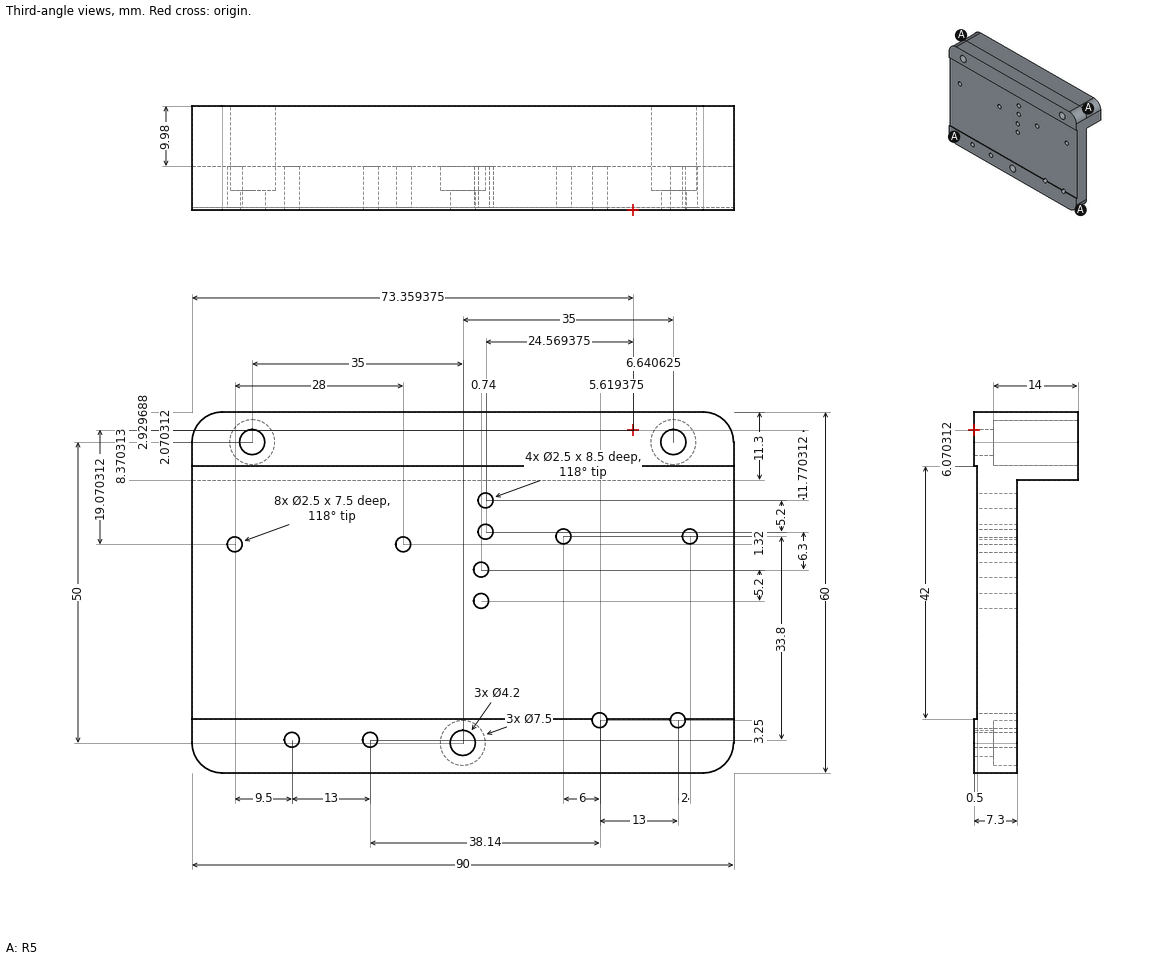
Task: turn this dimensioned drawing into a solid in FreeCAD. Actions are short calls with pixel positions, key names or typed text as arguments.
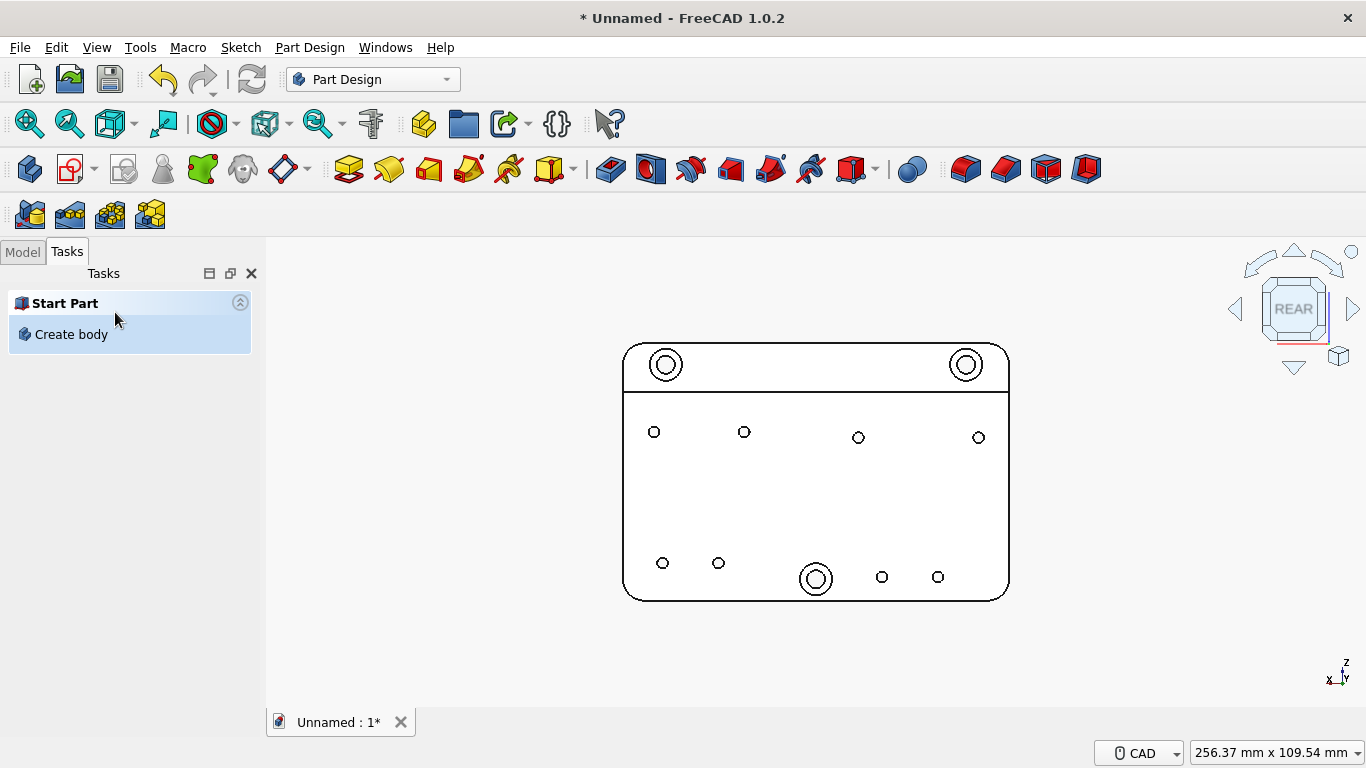
key(0)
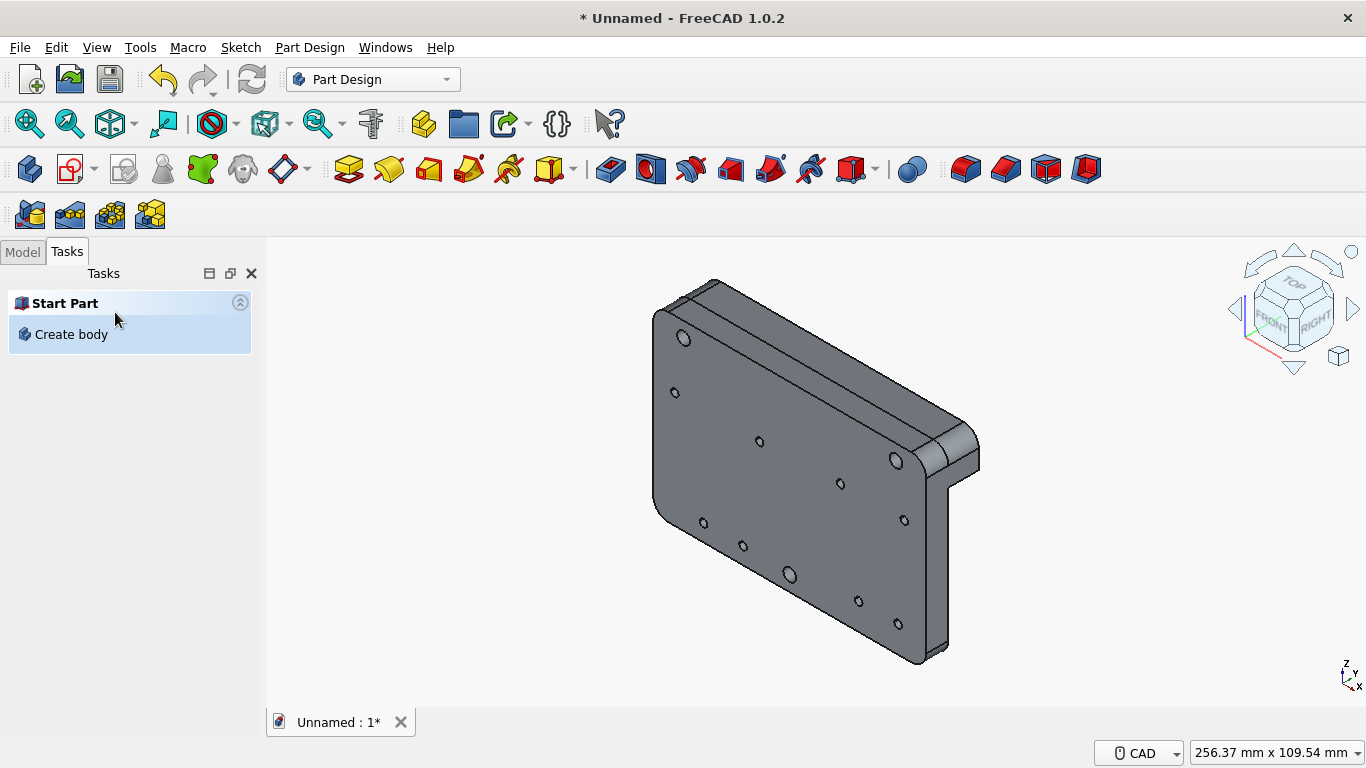
click(938, 508)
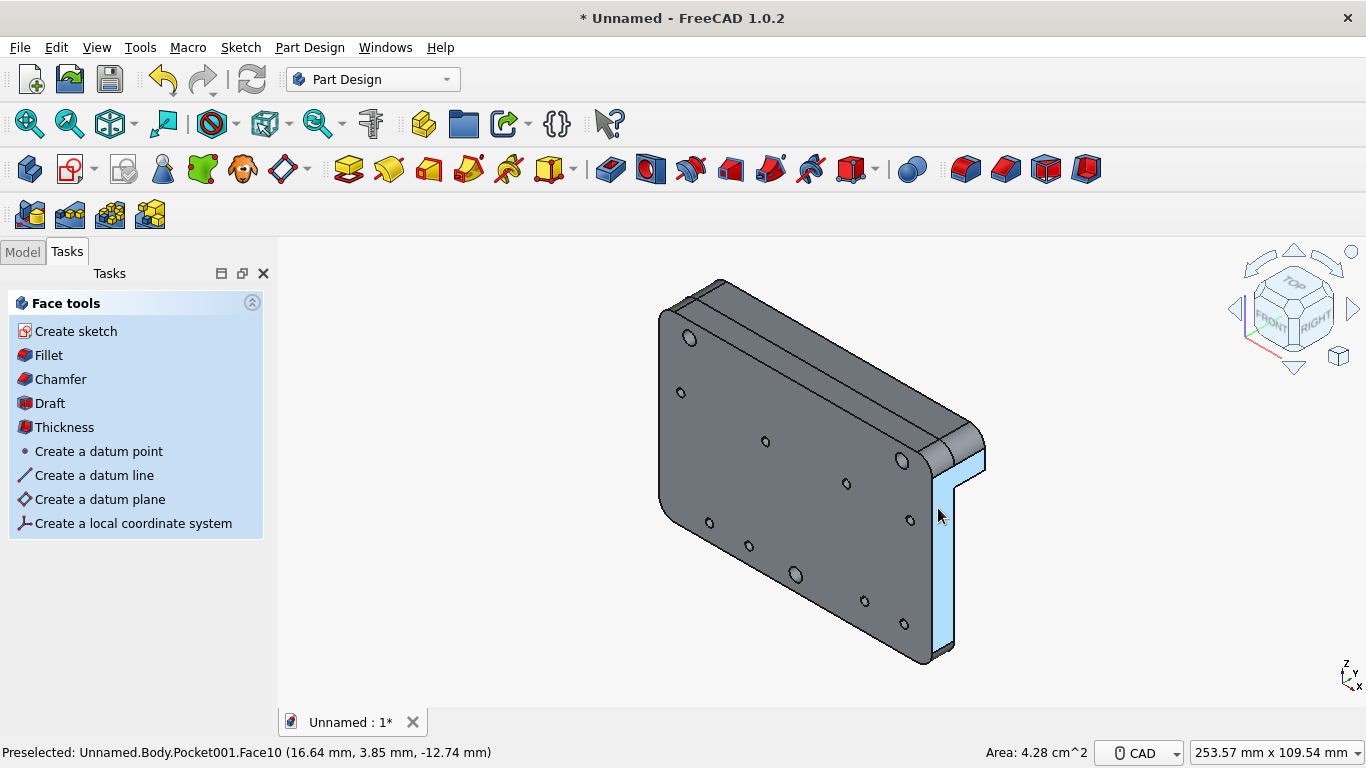
click(70, 170)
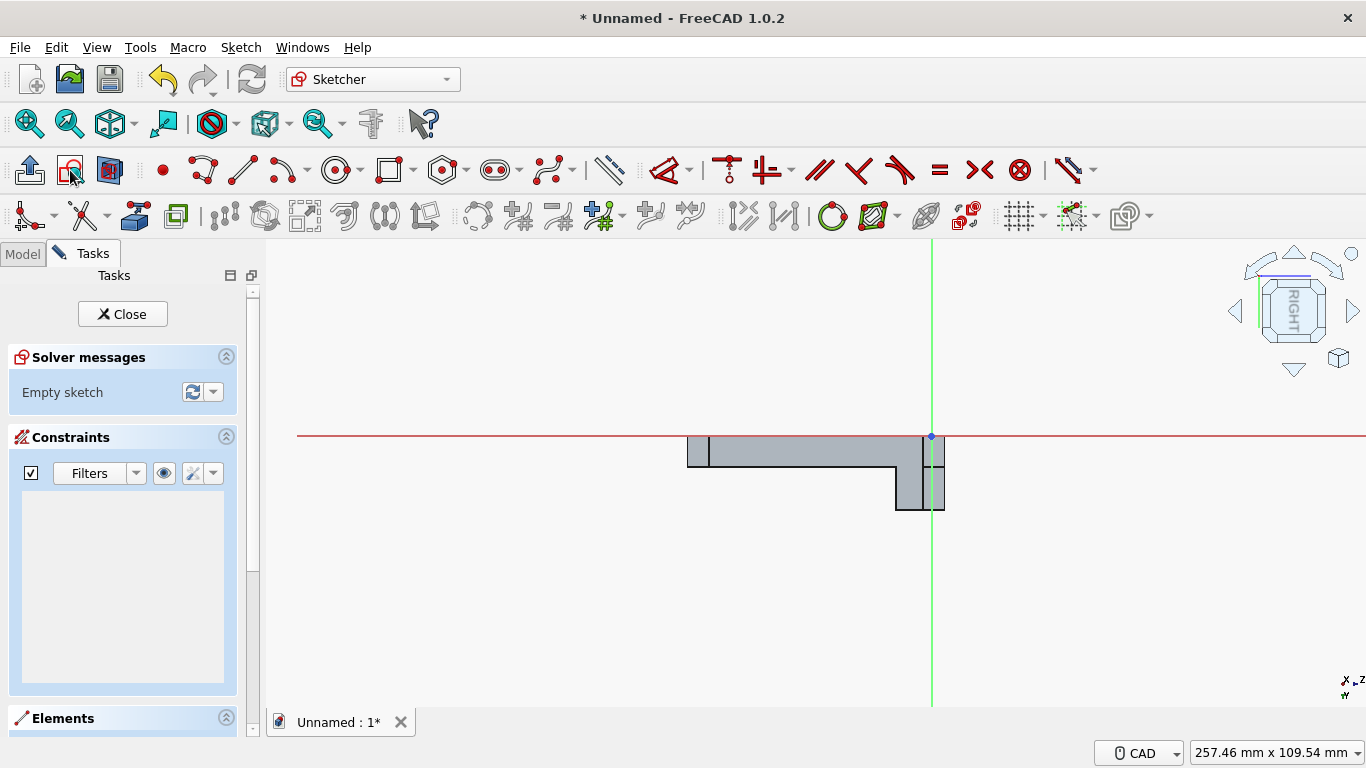
scroll(864, 422, up, 6)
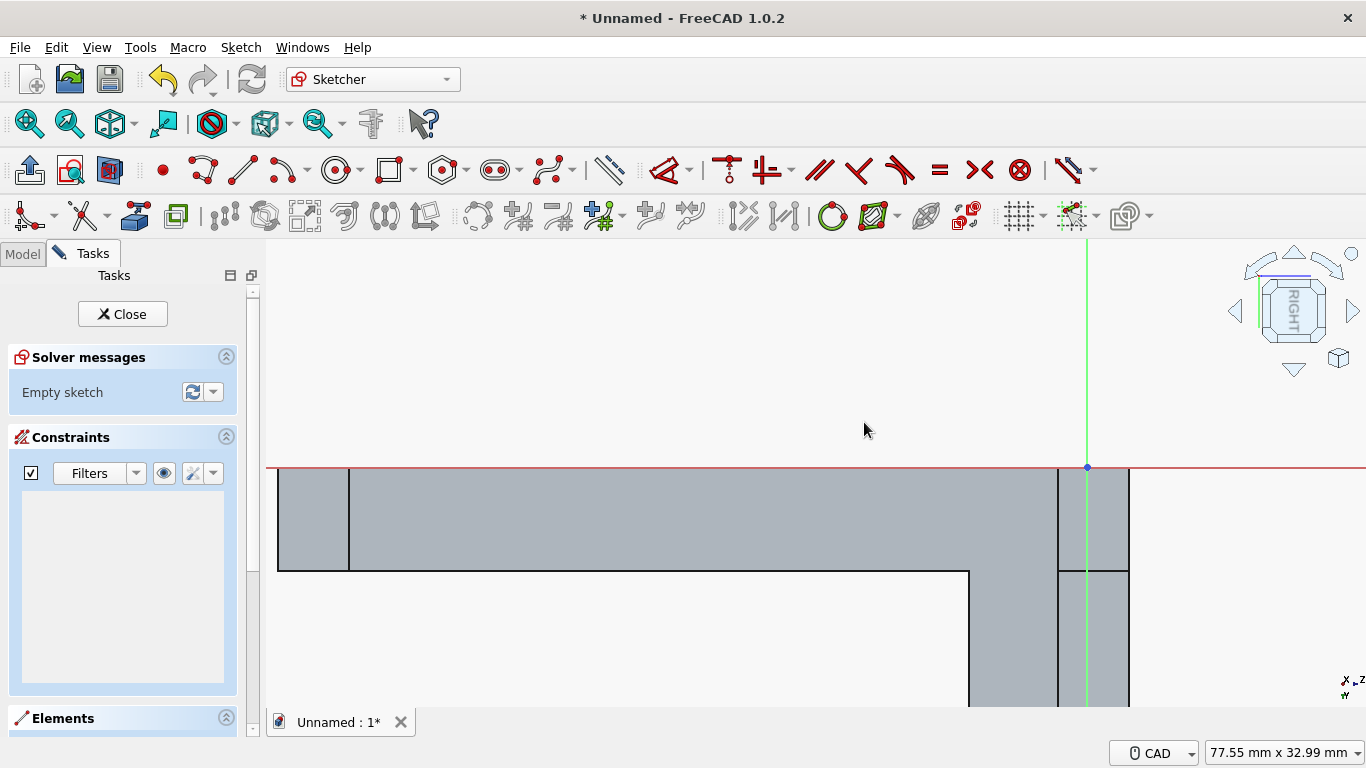
click(390, 170)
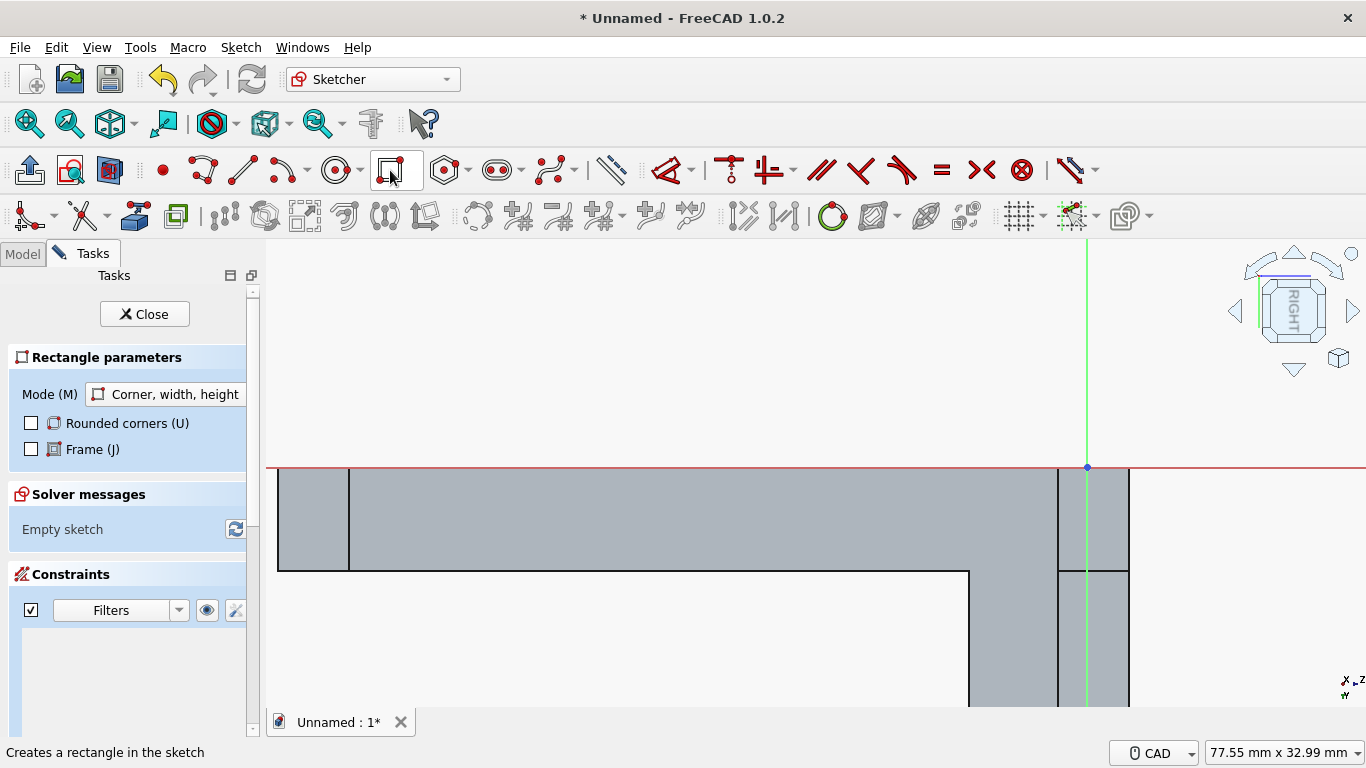
scroll(405, 468, up, 5)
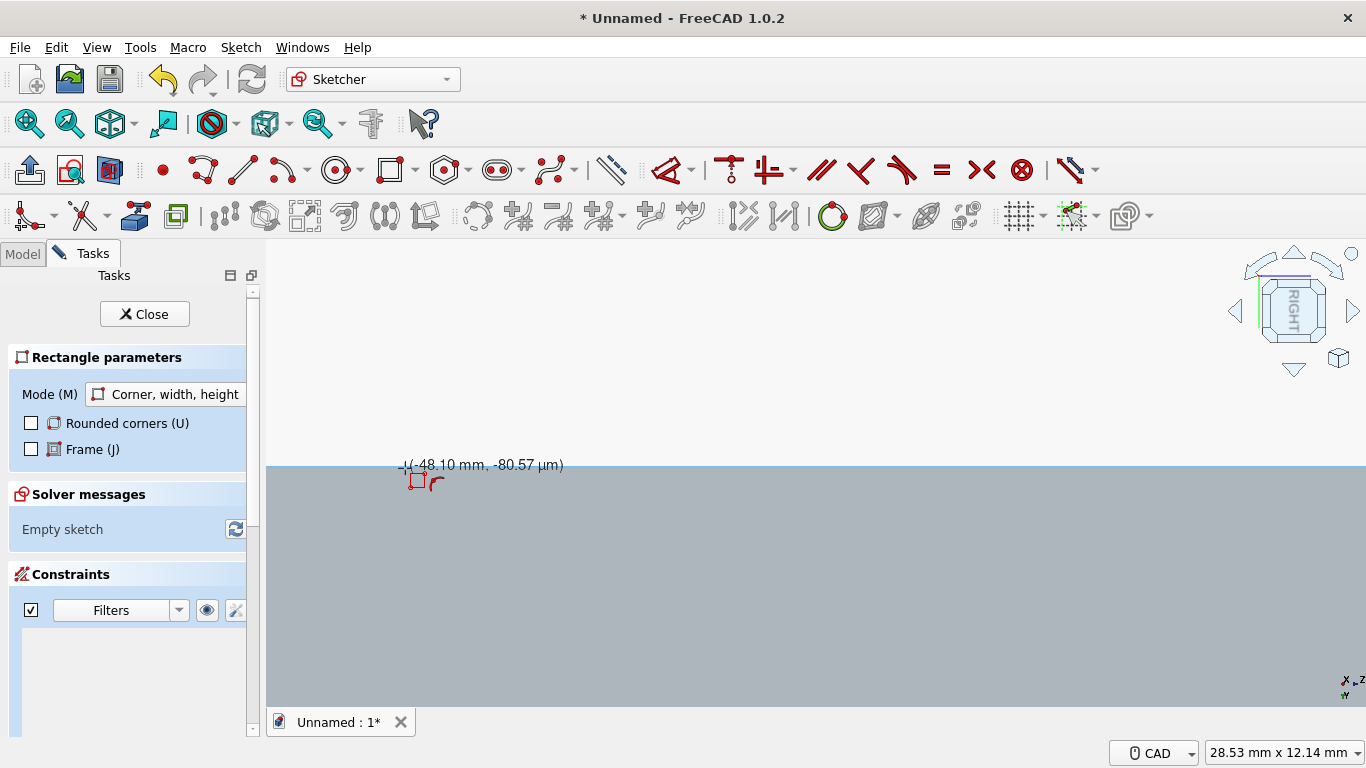
click(406, 467)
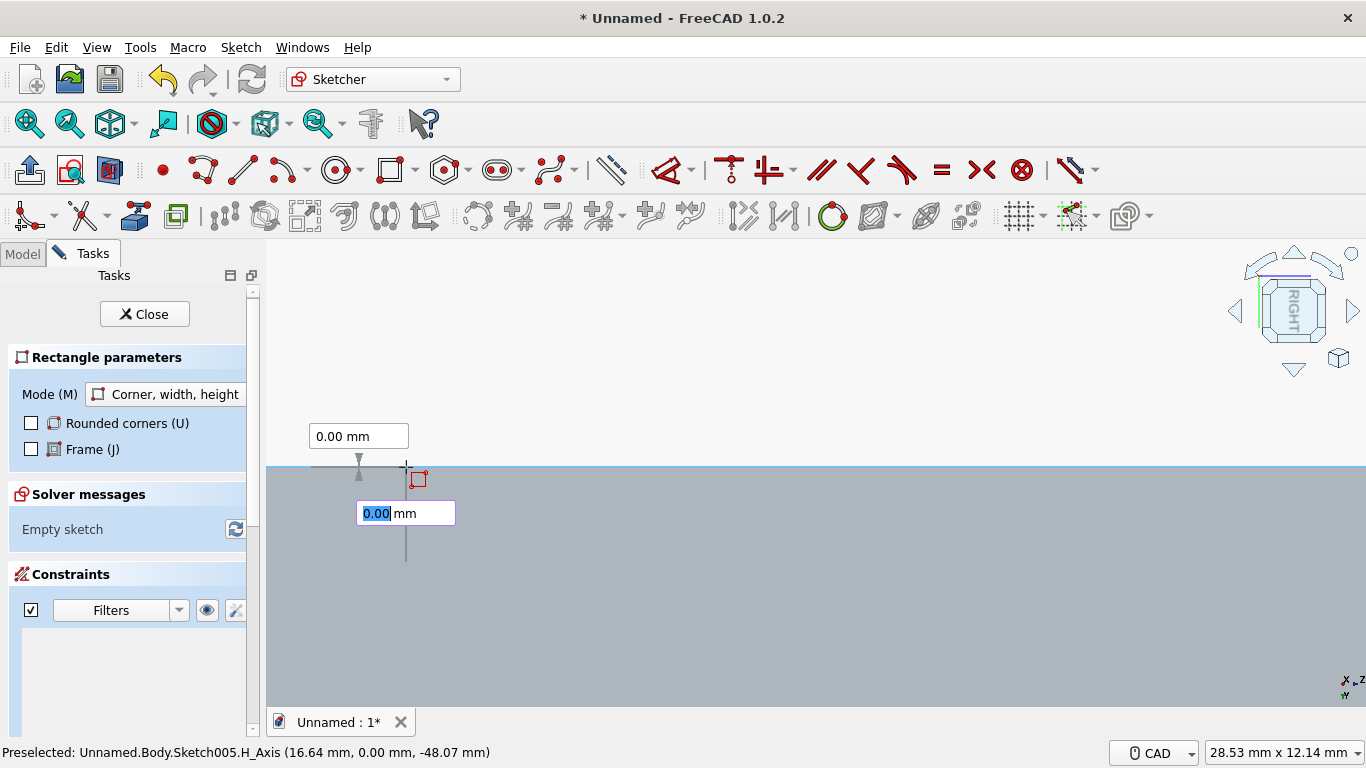
scroll(407, 471, down, 5)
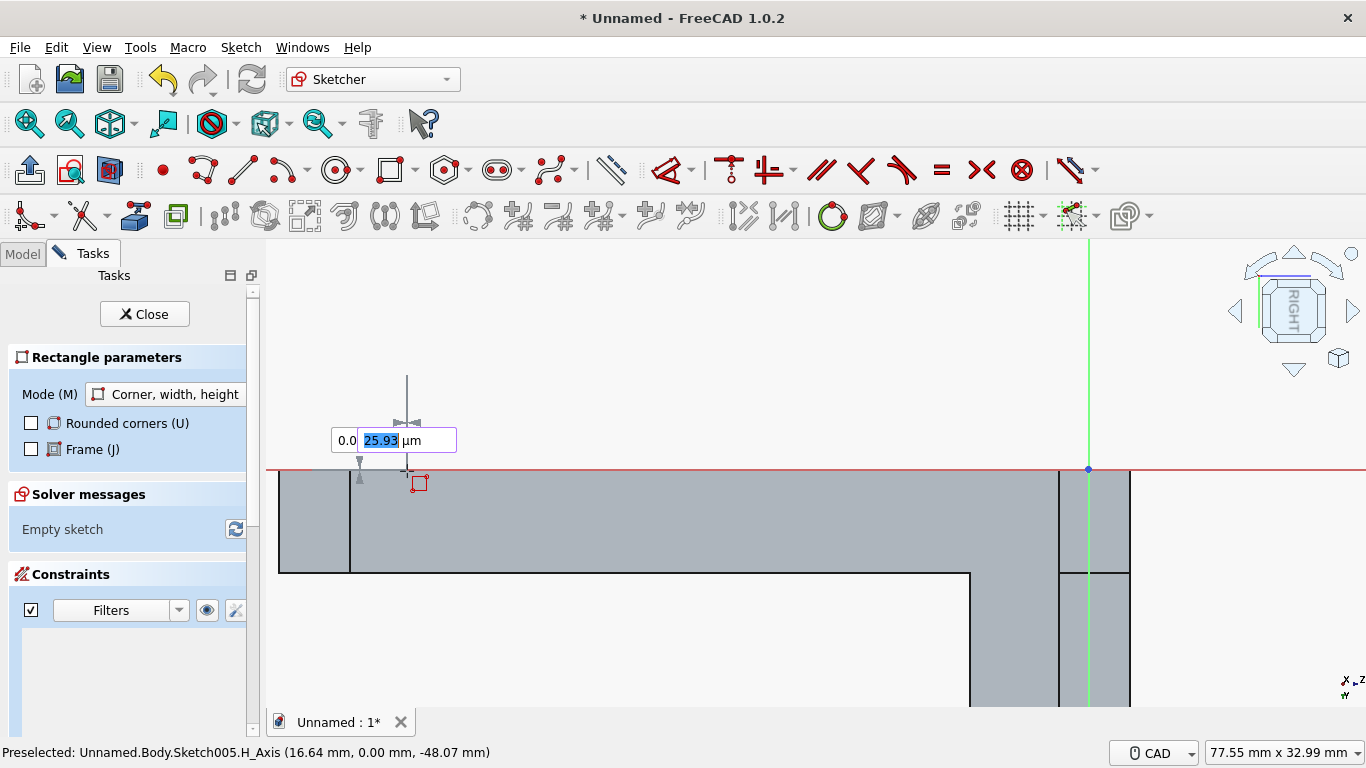
scroll(1003, 477, up, 5)